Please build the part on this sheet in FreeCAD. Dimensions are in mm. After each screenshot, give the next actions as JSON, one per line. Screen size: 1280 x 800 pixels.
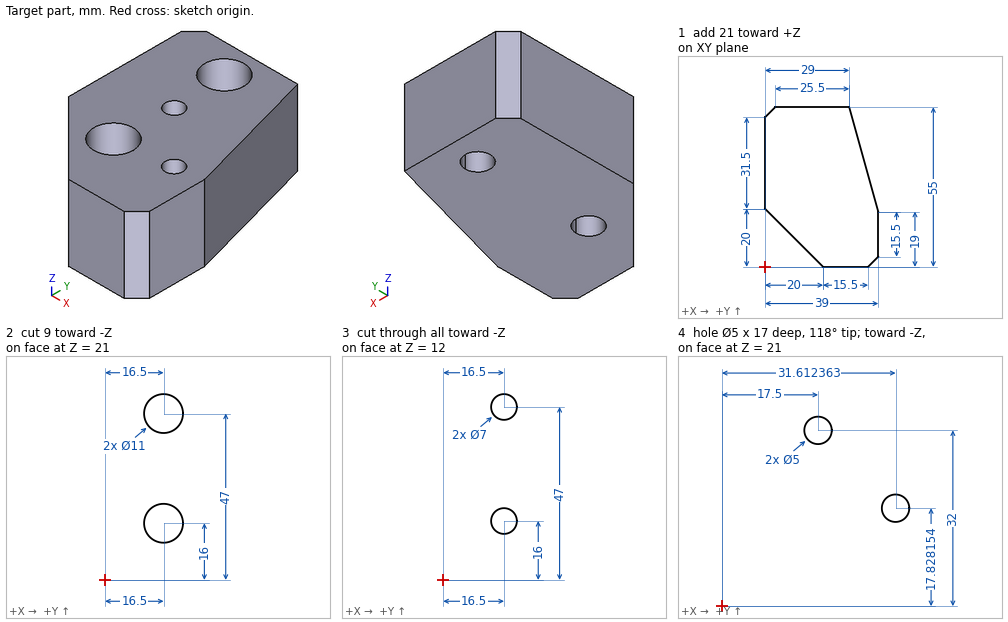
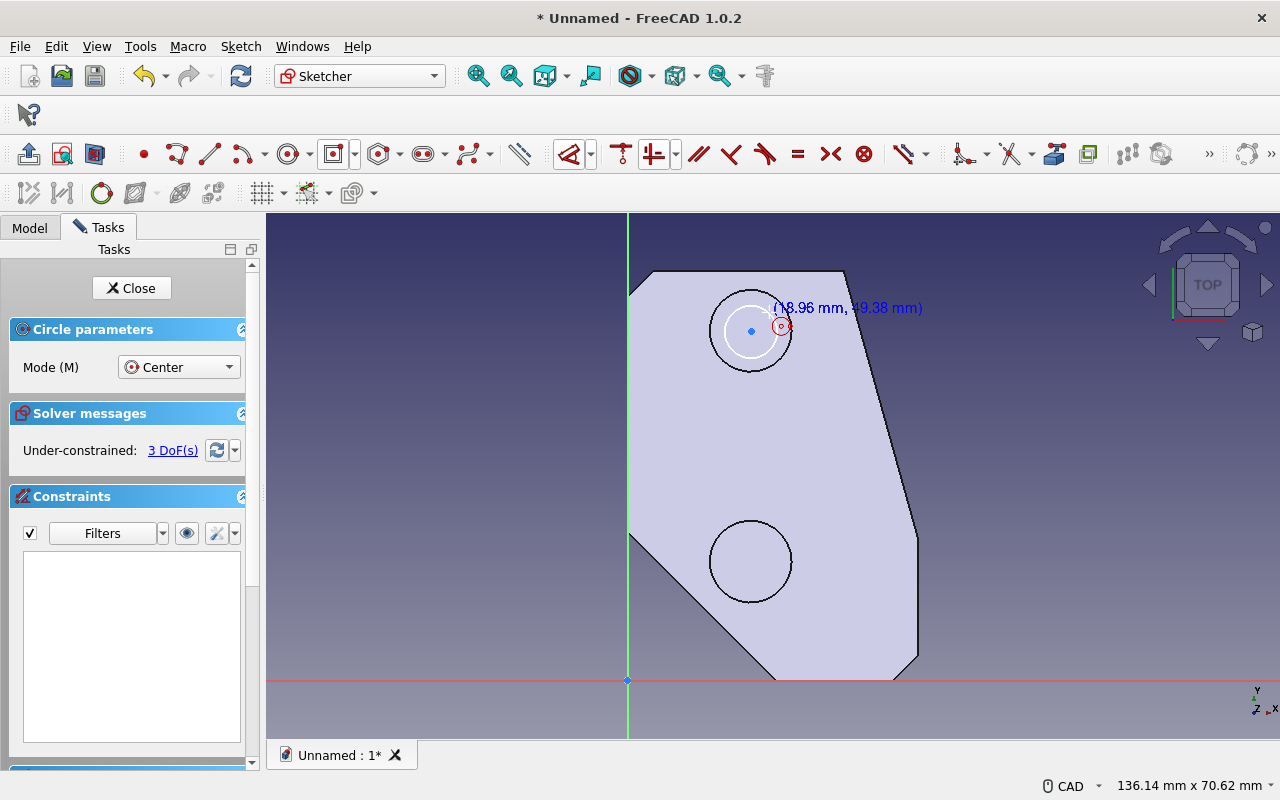
{"action": "left_click", "coordinate": [751, 562]}
{"action": "left_click", "coordinate": [769, 543]}
{"action": "key", "text": "Escape"}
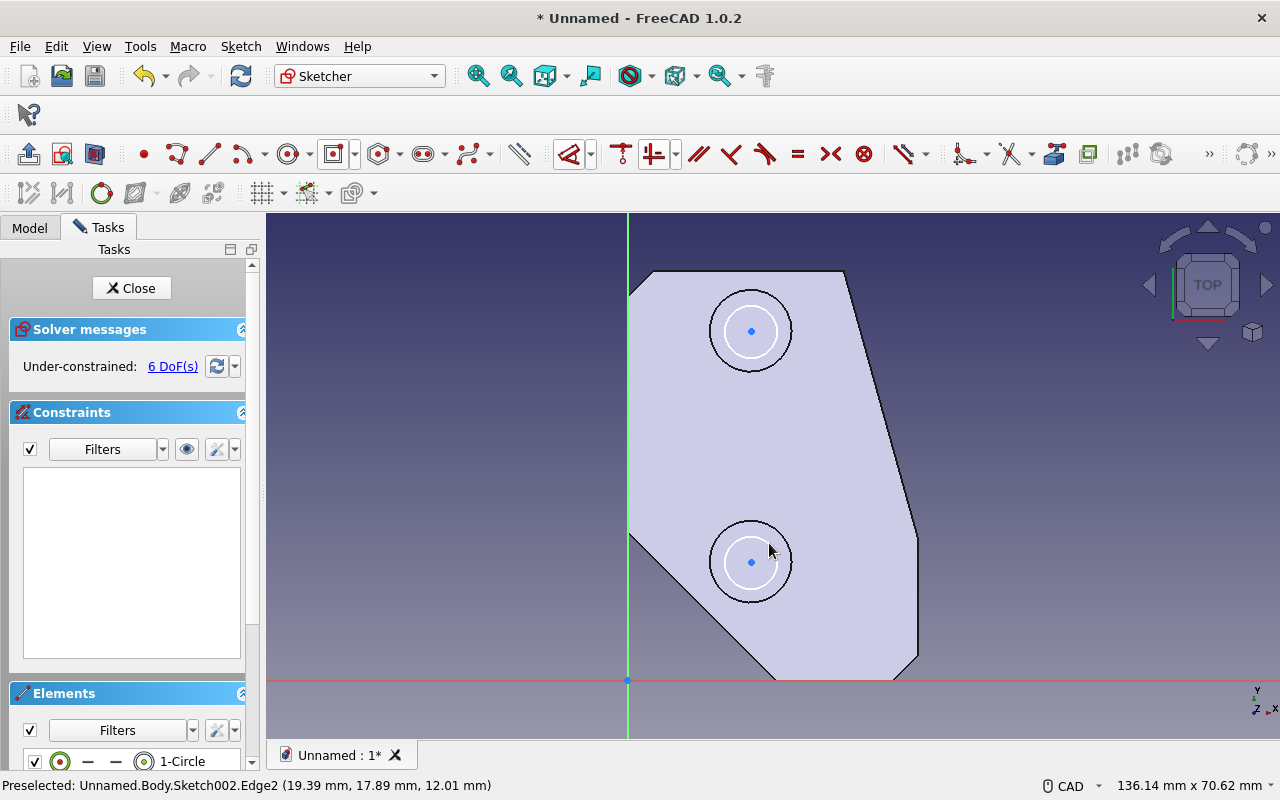
{"action": "left_click", "coordinate": [769, 313]}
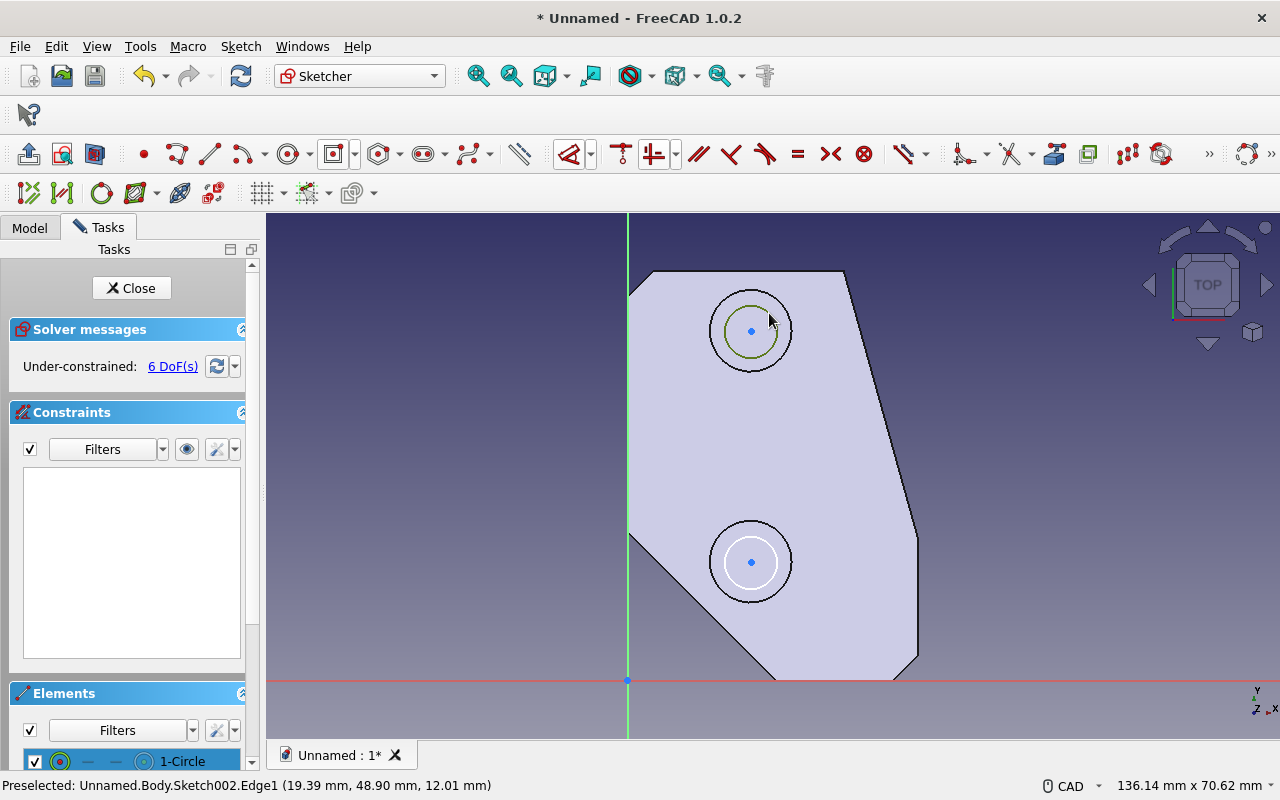
{"action": "left_click", "coordinate": [769, 544]}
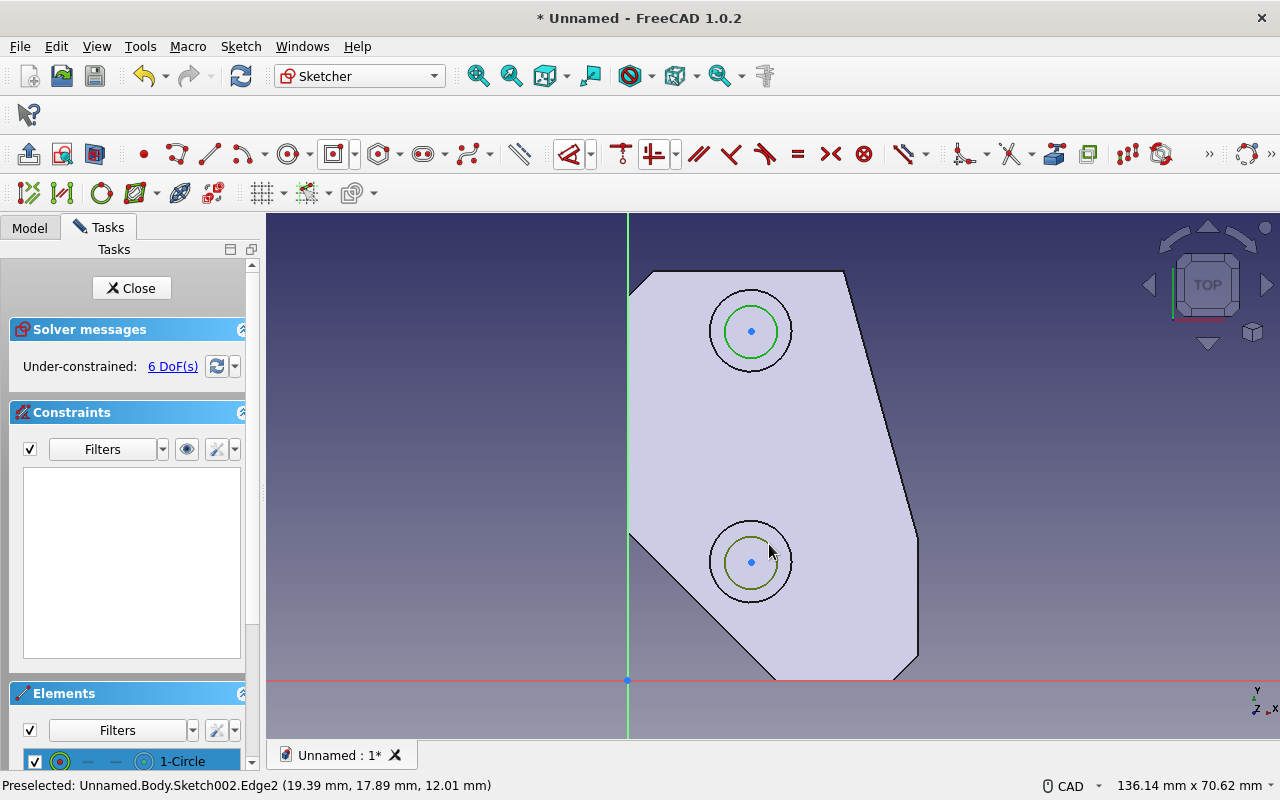
{"action": "left_click", "coordinate": [798, 154]}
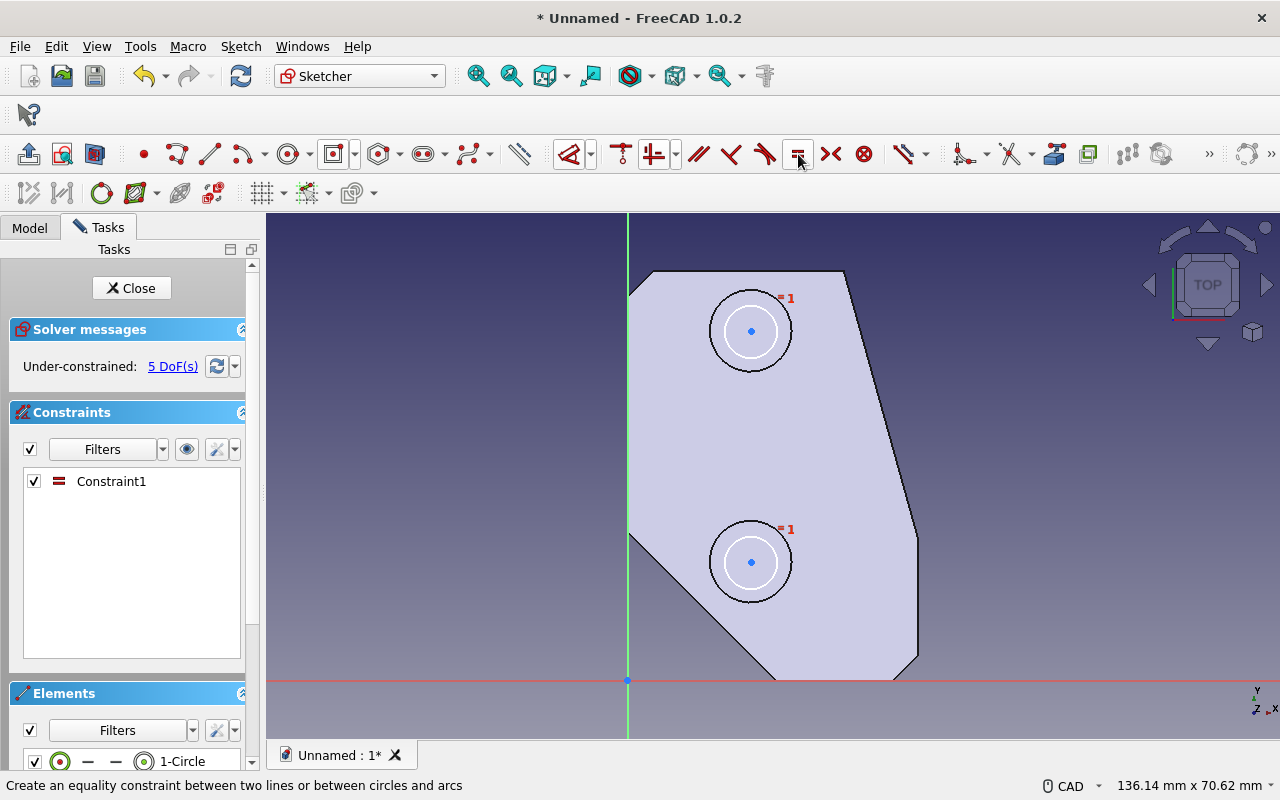
{"action": "left_click", "coordinate": [769, 313]}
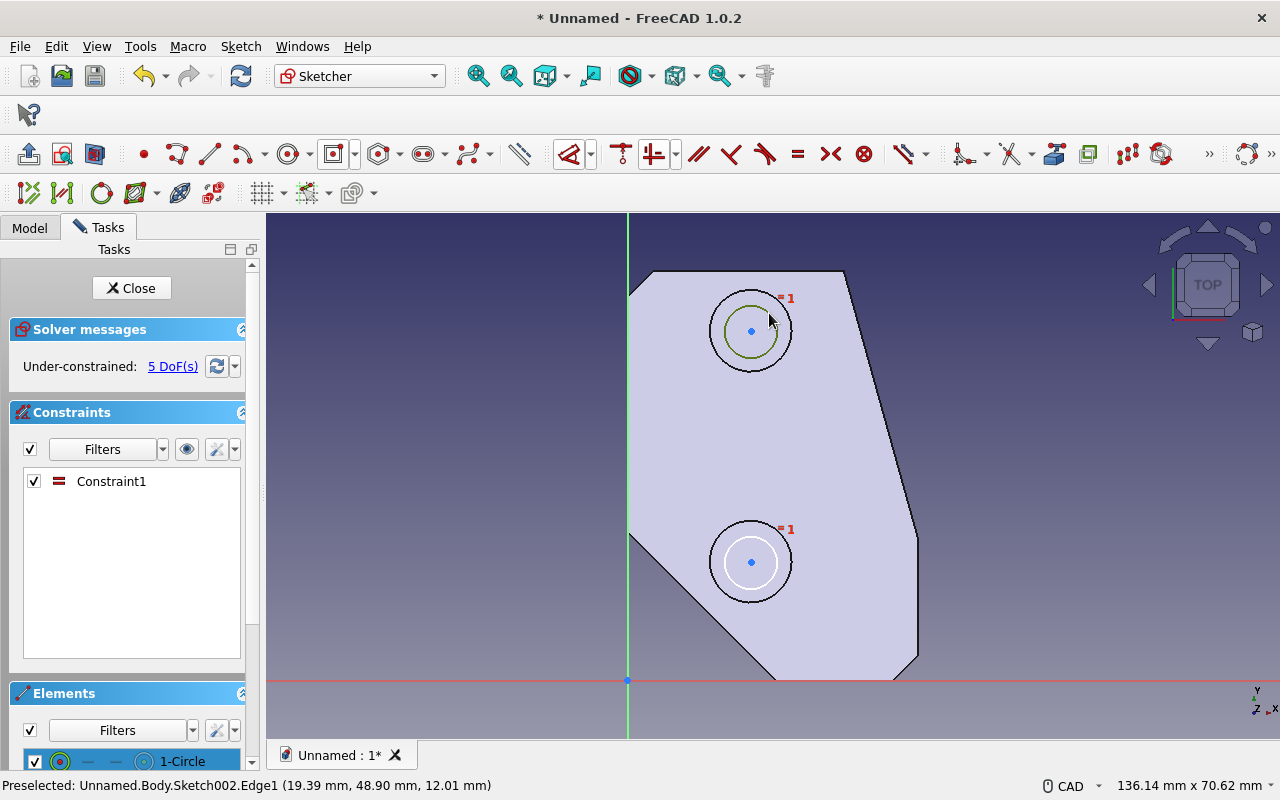
{"action": "left_click", "coordinate": [590, 154]}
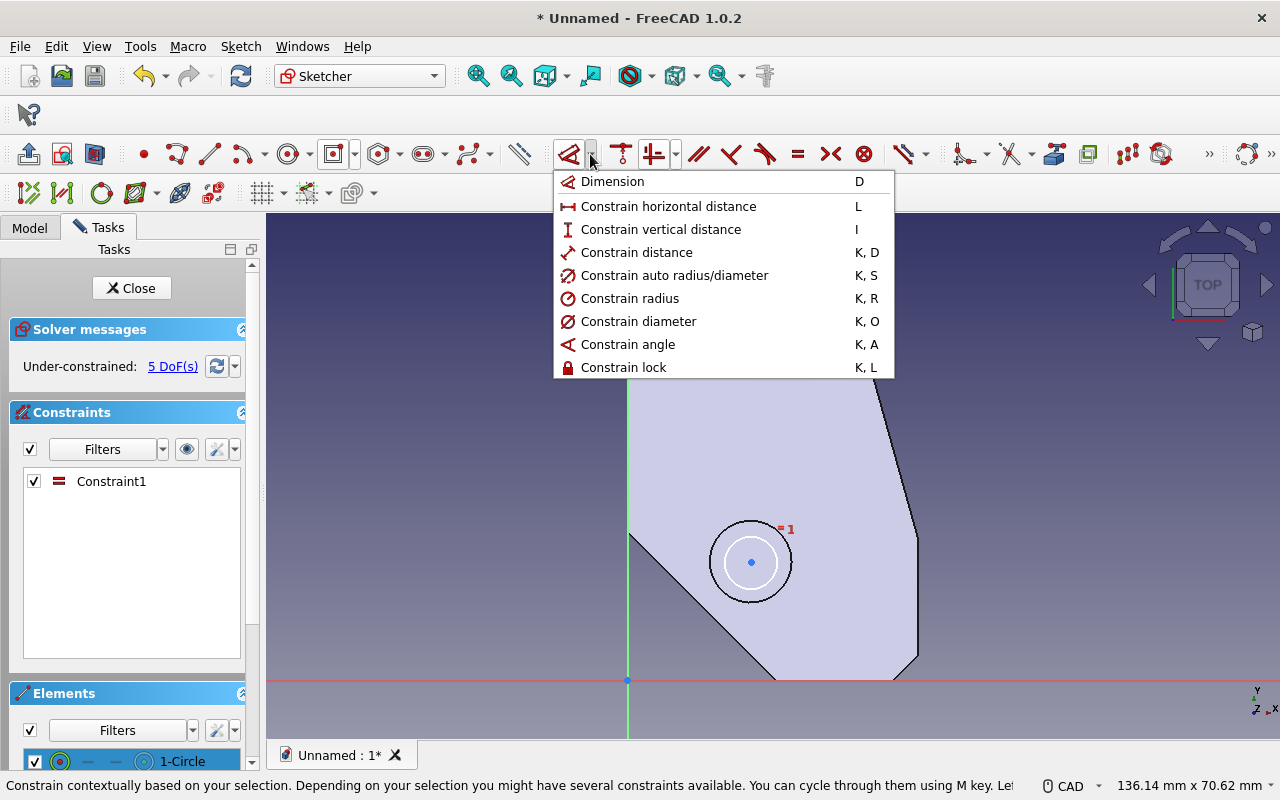
{"action": "left_click", "coordinate": [724, 322]}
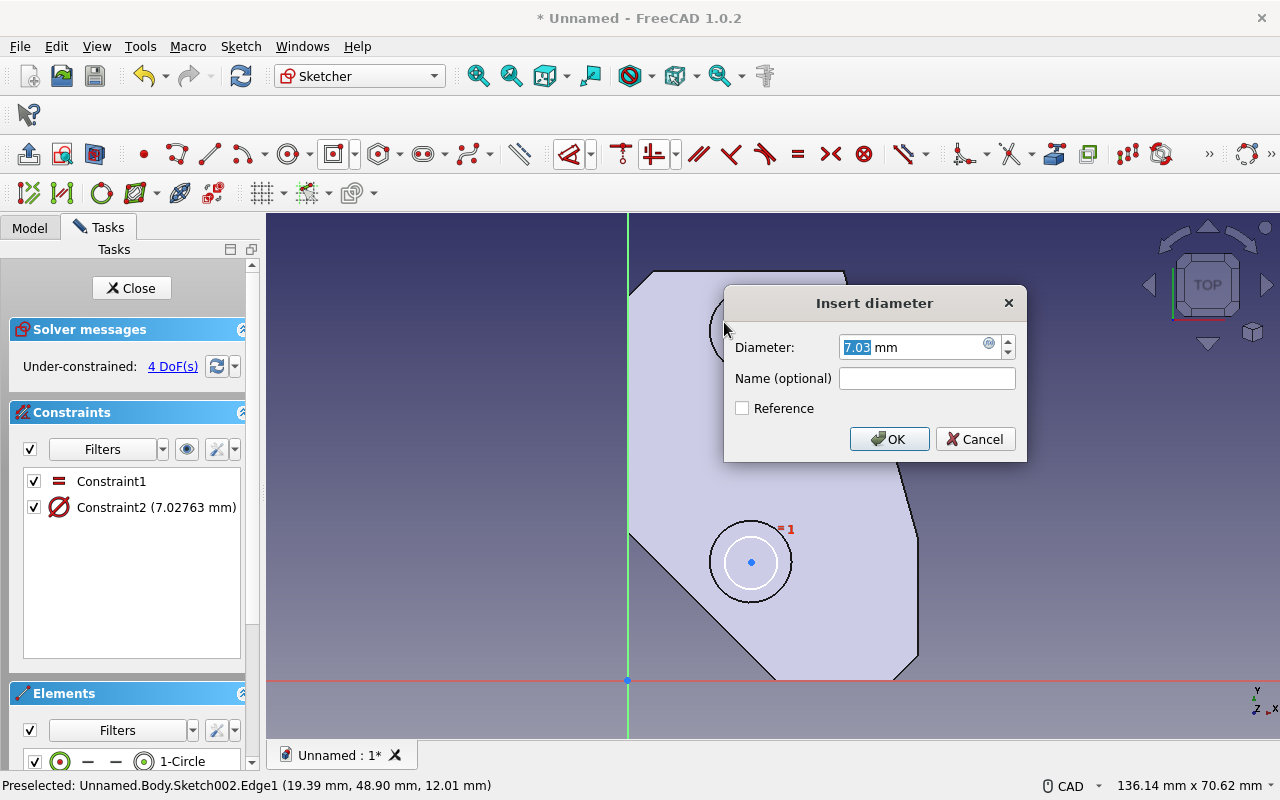
{"action": "type", "text": "7"}
{"action": "key", "text": "Return"}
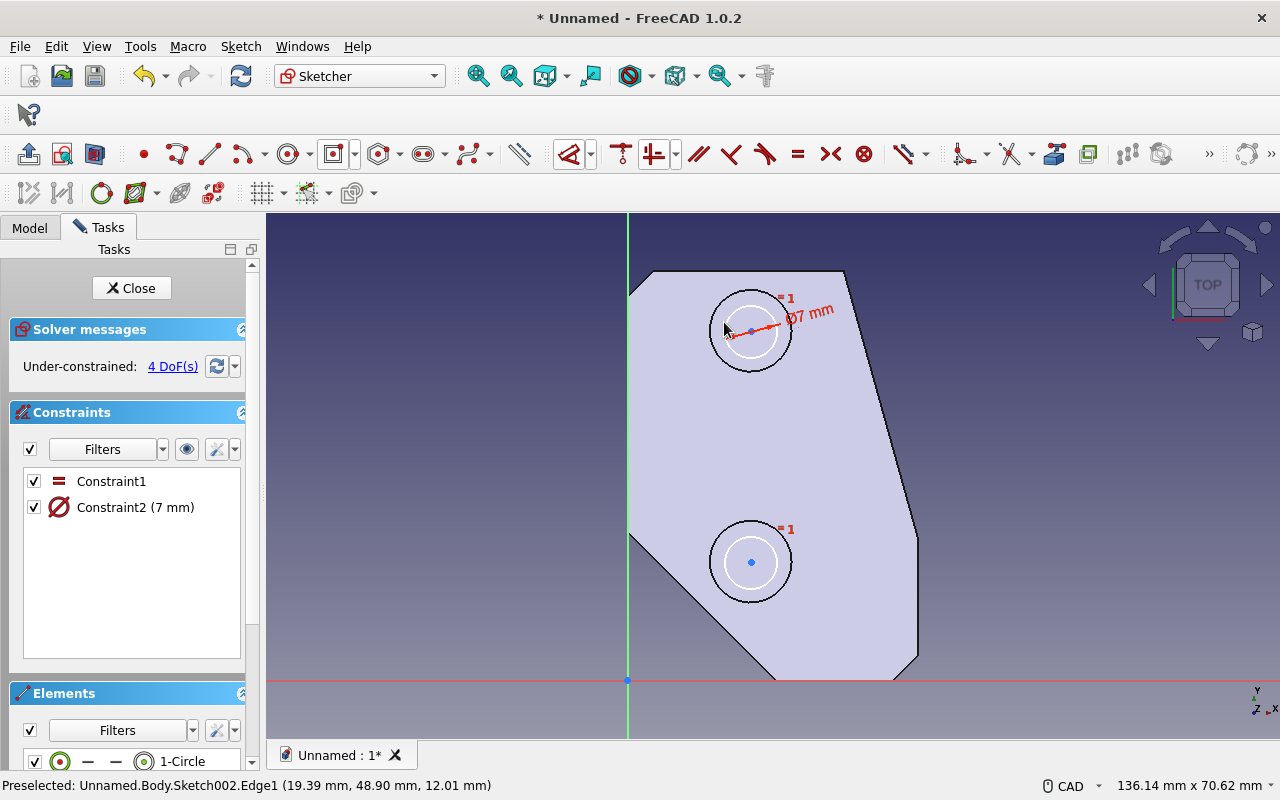
{"action": "left_click", "coordinate": [751, 332]}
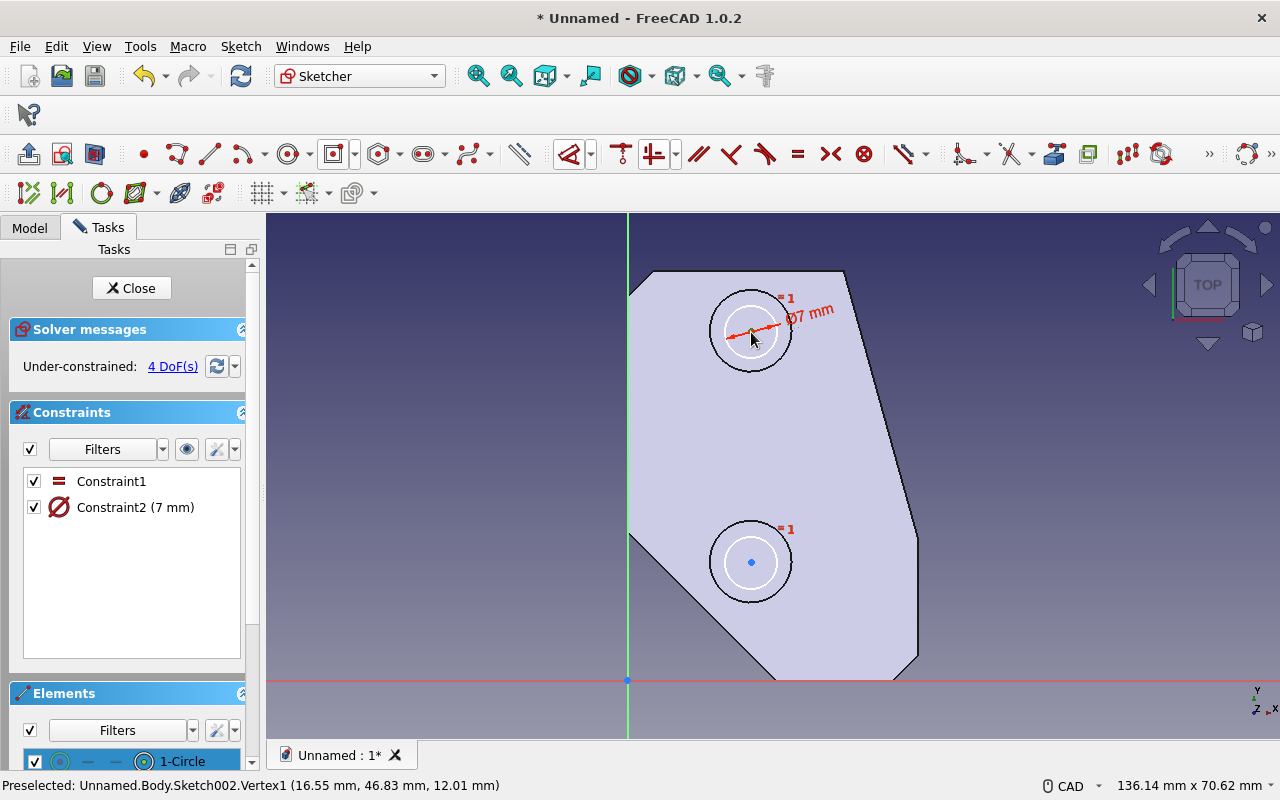
{"action": "key", "text": "i"}